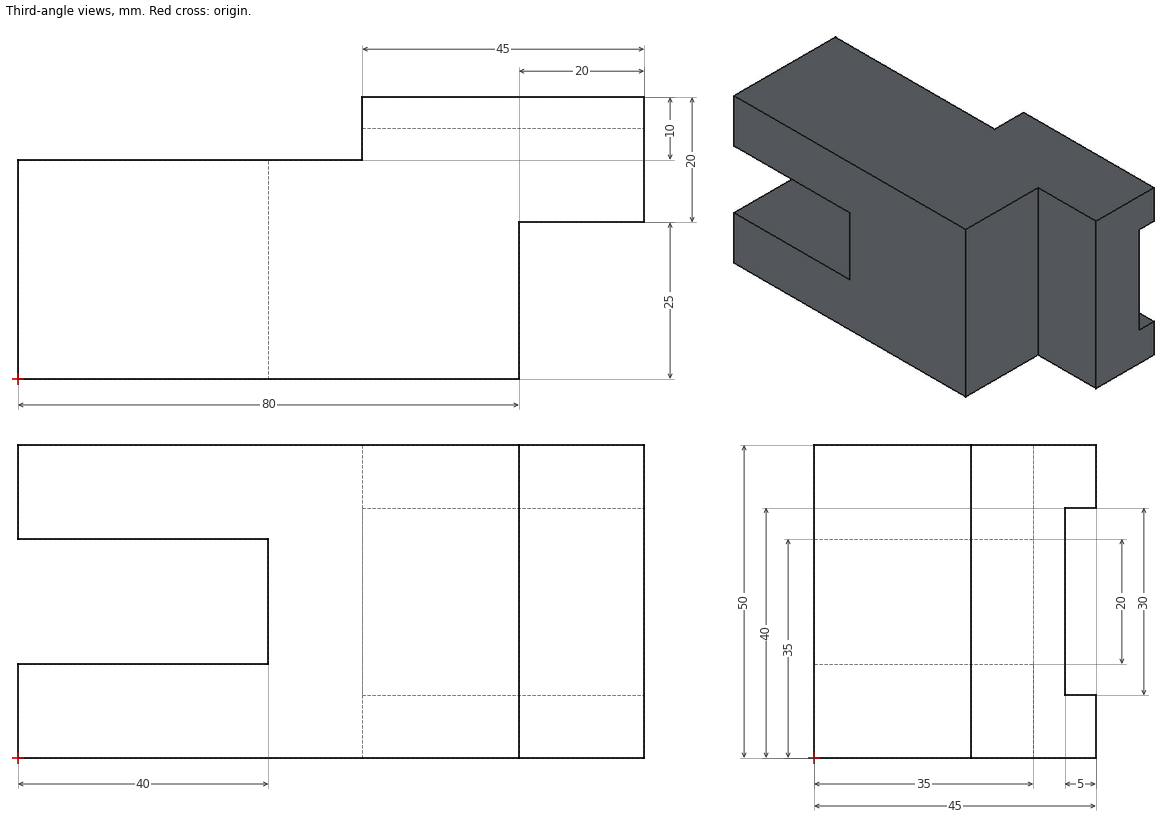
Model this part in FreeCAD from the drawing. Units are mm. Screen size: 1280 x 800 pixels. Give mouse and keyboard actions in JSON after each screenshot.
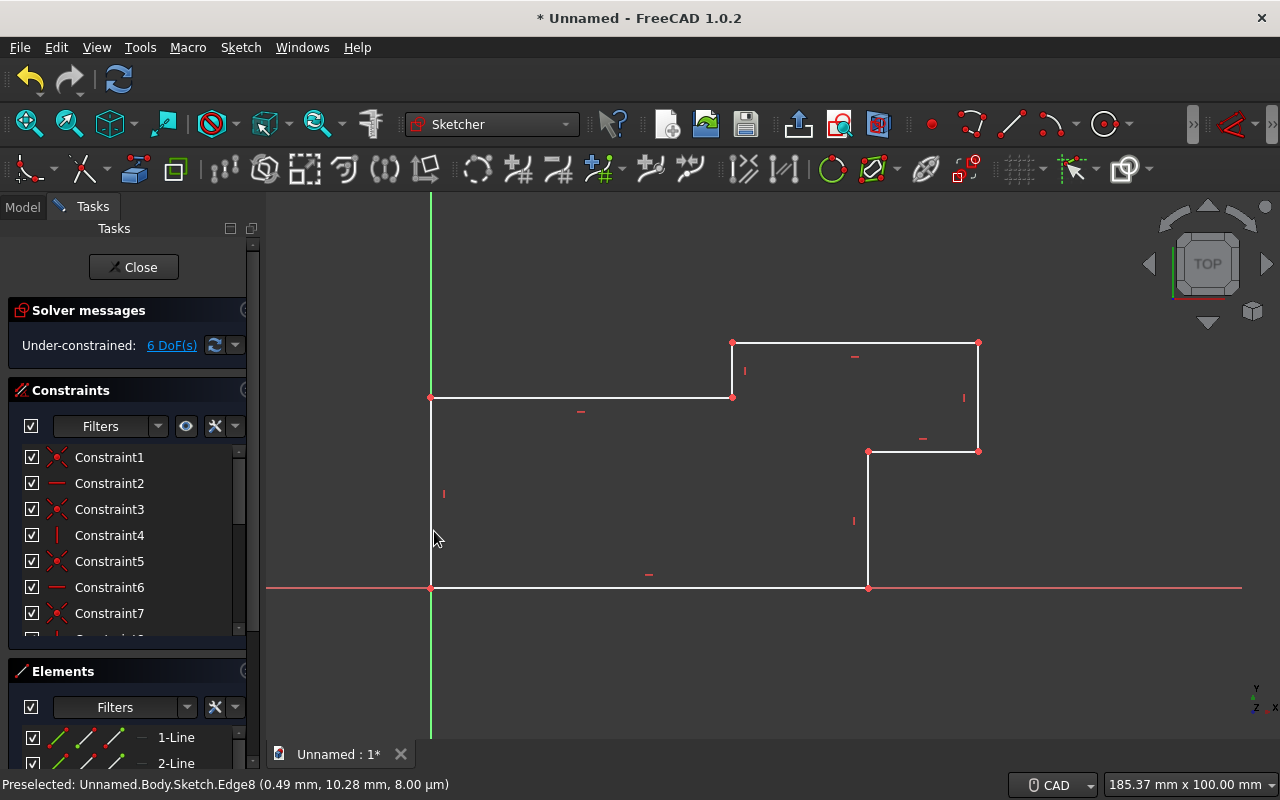
{"action": "left_click", "coordinate": [1232, 124]}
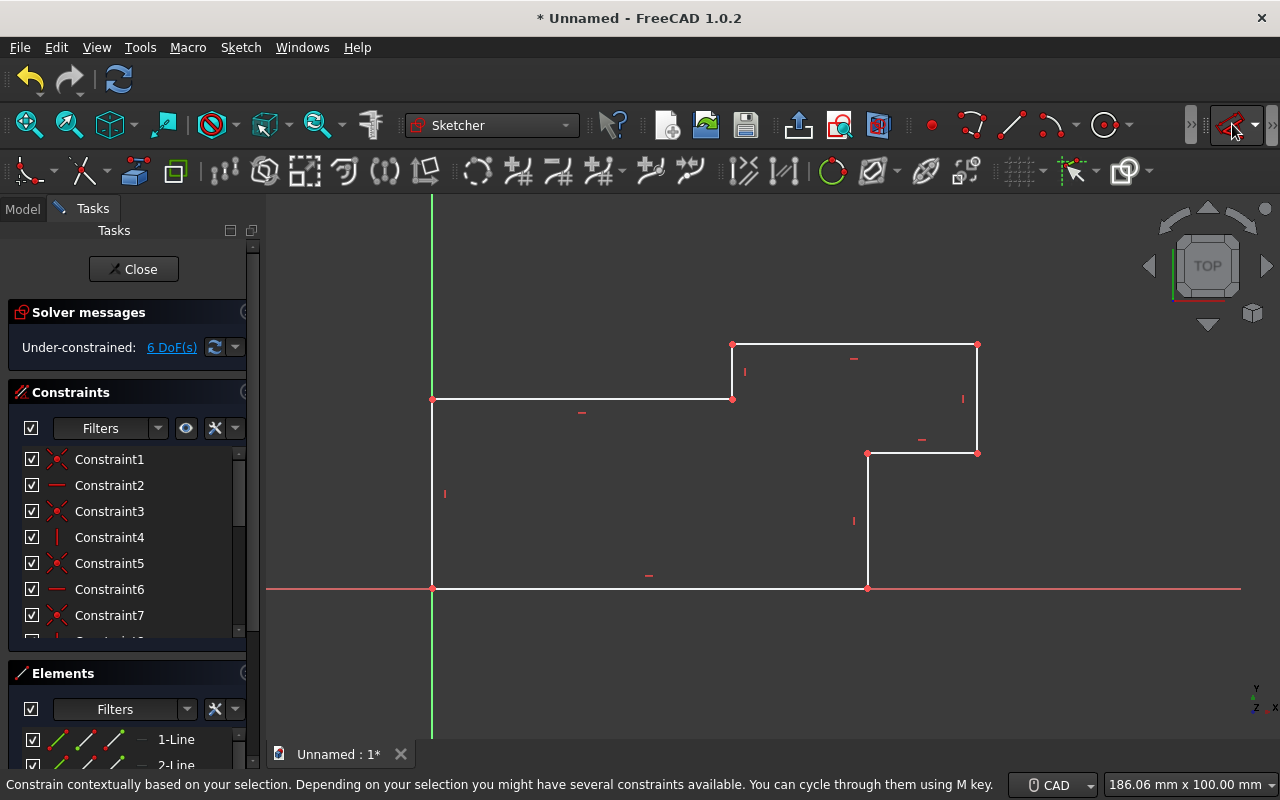
{"action": "left_click", "coordinate": [563, 589]}
{"action": "left_click", "coordinate": [650, 623]}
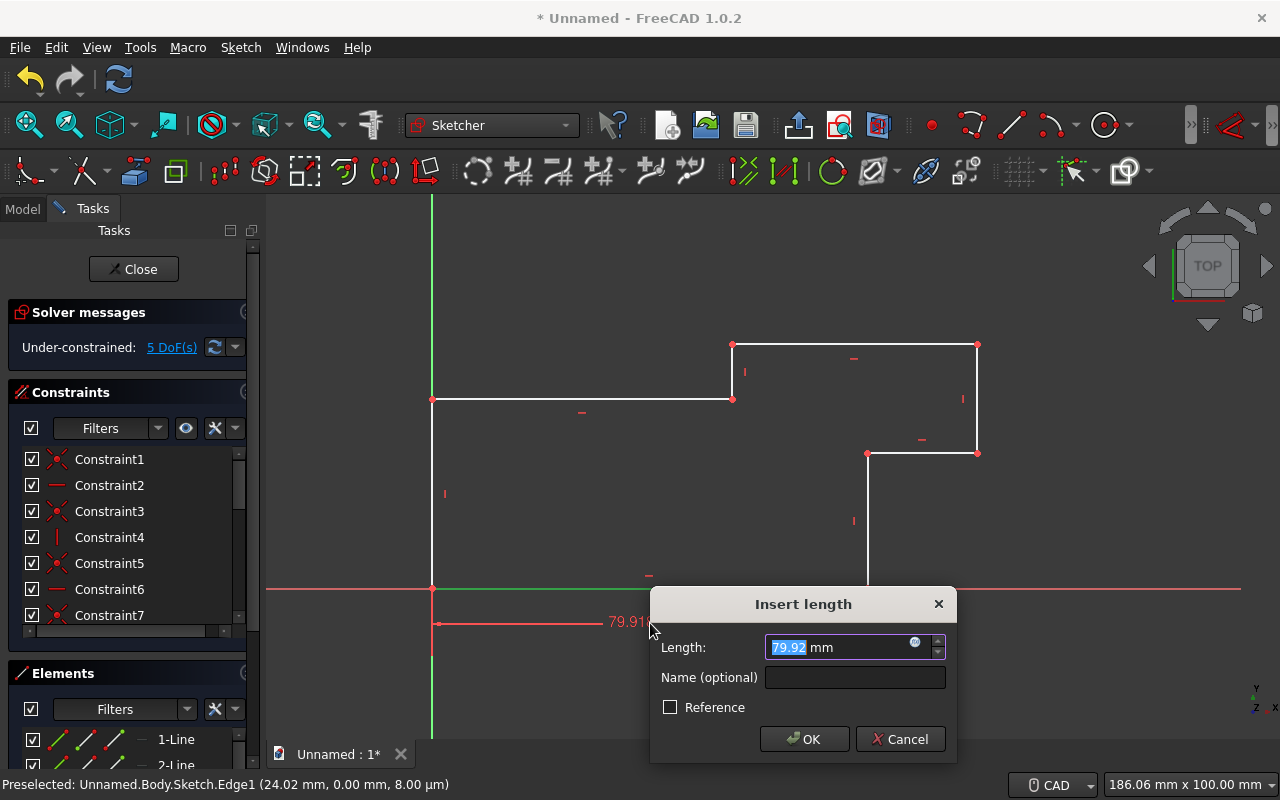
{"action": "type", "text": "80"}
{"action": "key", "text": "Return"}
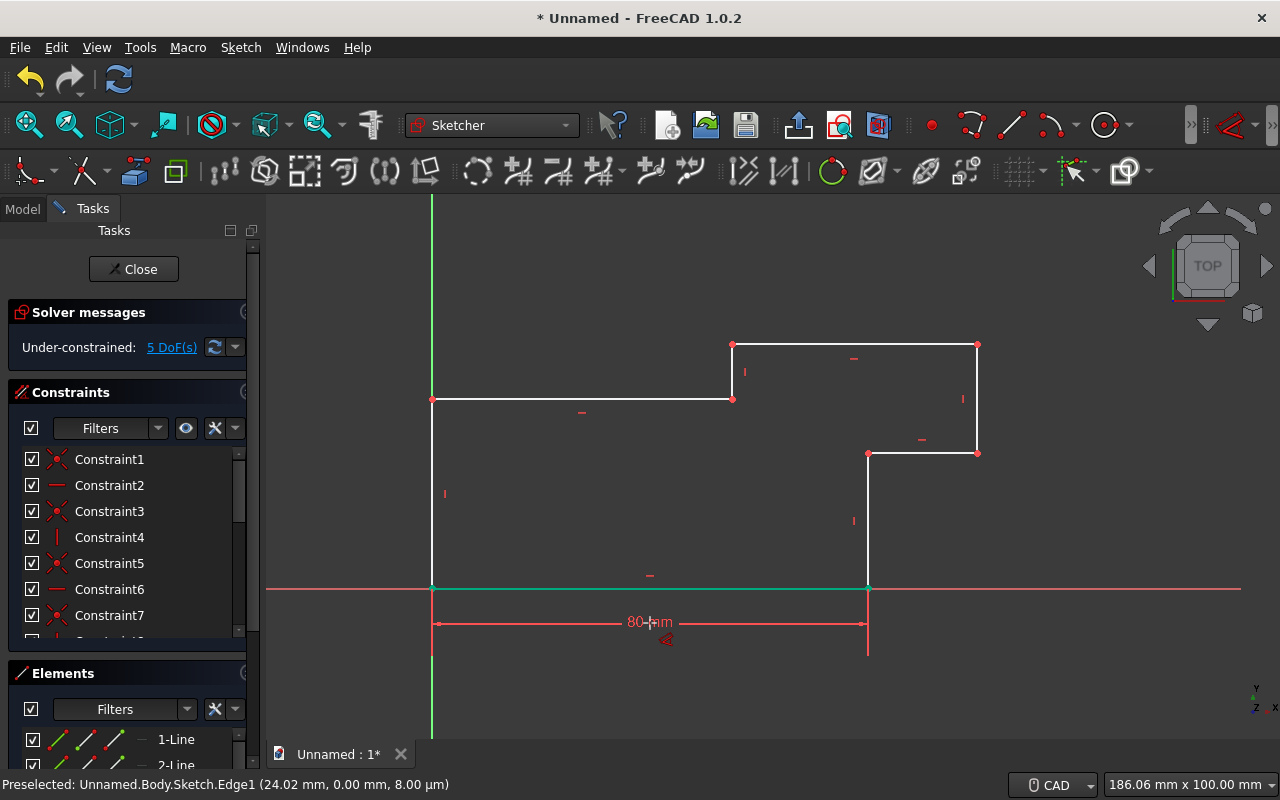
{"action": "left_click", "coordinate": [868, 548]}
{"action": "left_click", "coordinate": [902, 521]}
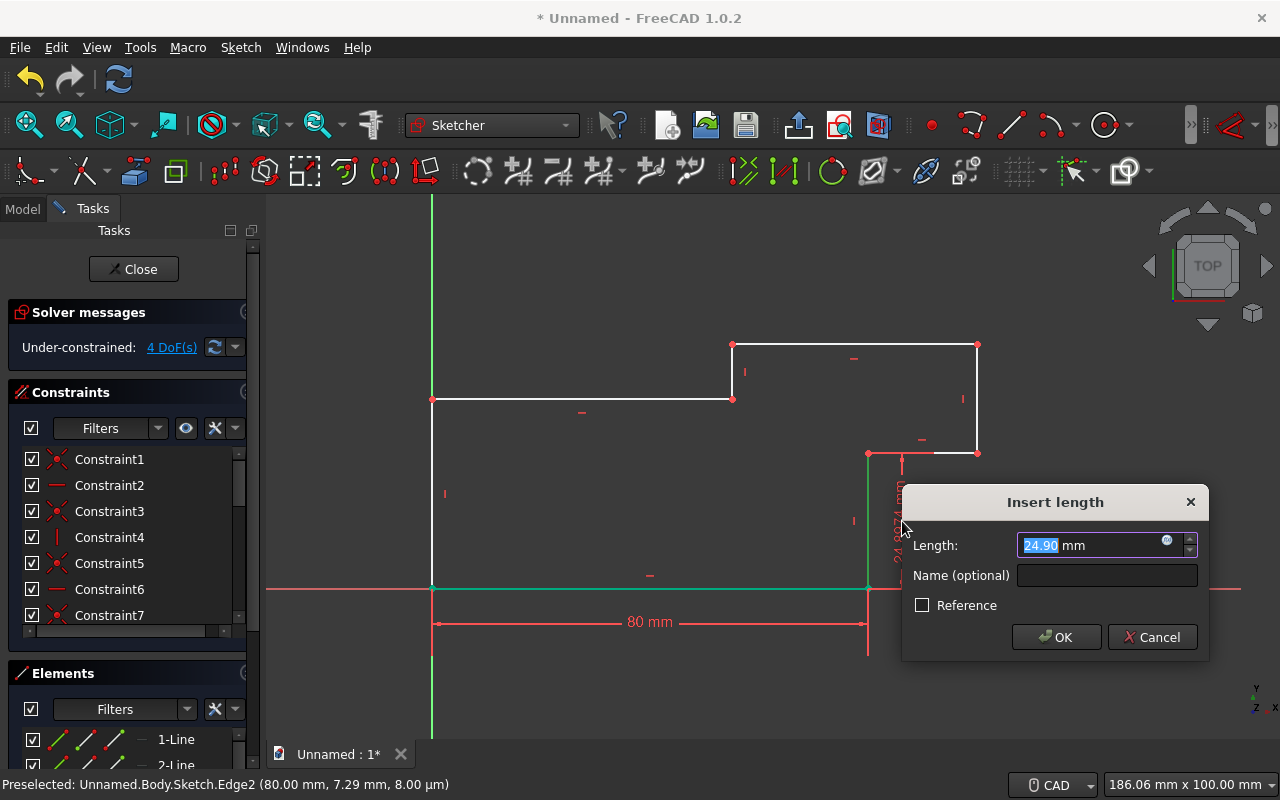
{"action": "type", "text": "25"}
{"action": "key", "text": "Return"}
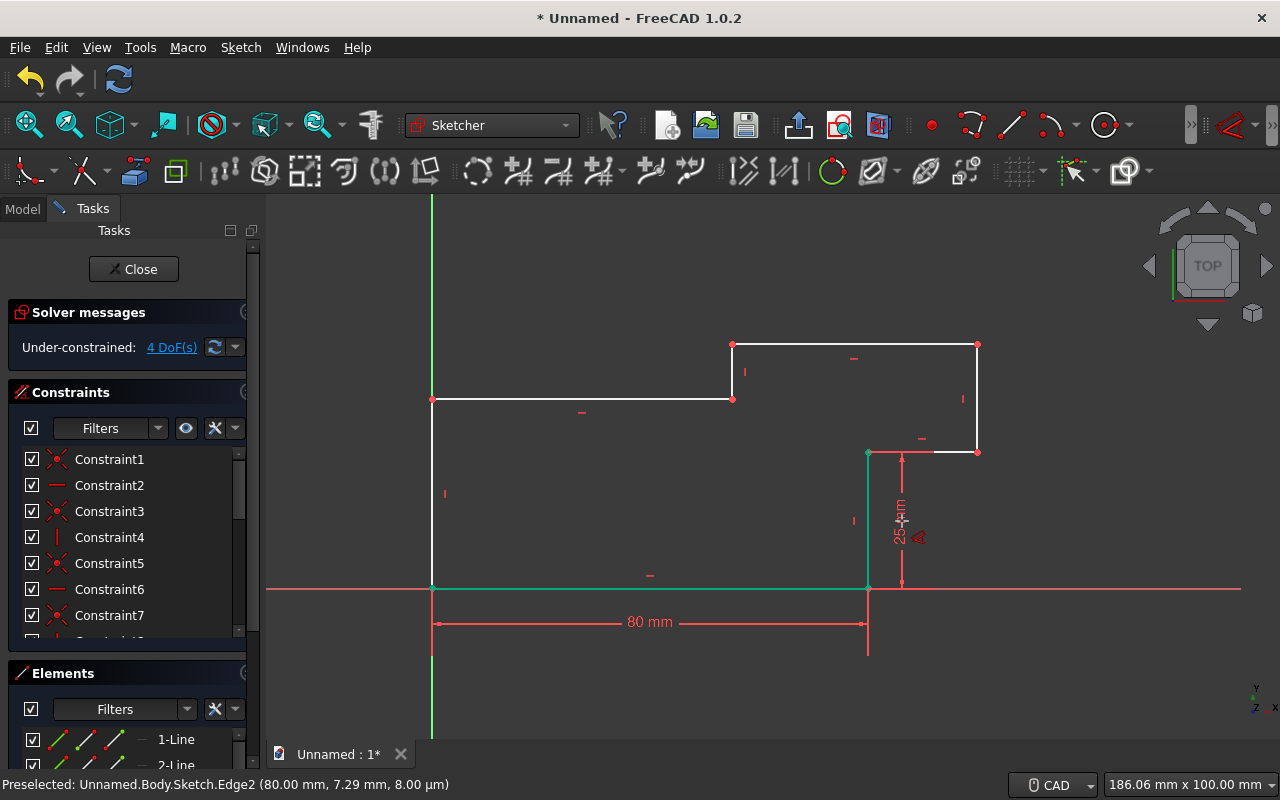
{"action": "left_click", "coordinate": [901, 452]}
{"action": "left_click", "coordinate": [923, 418]}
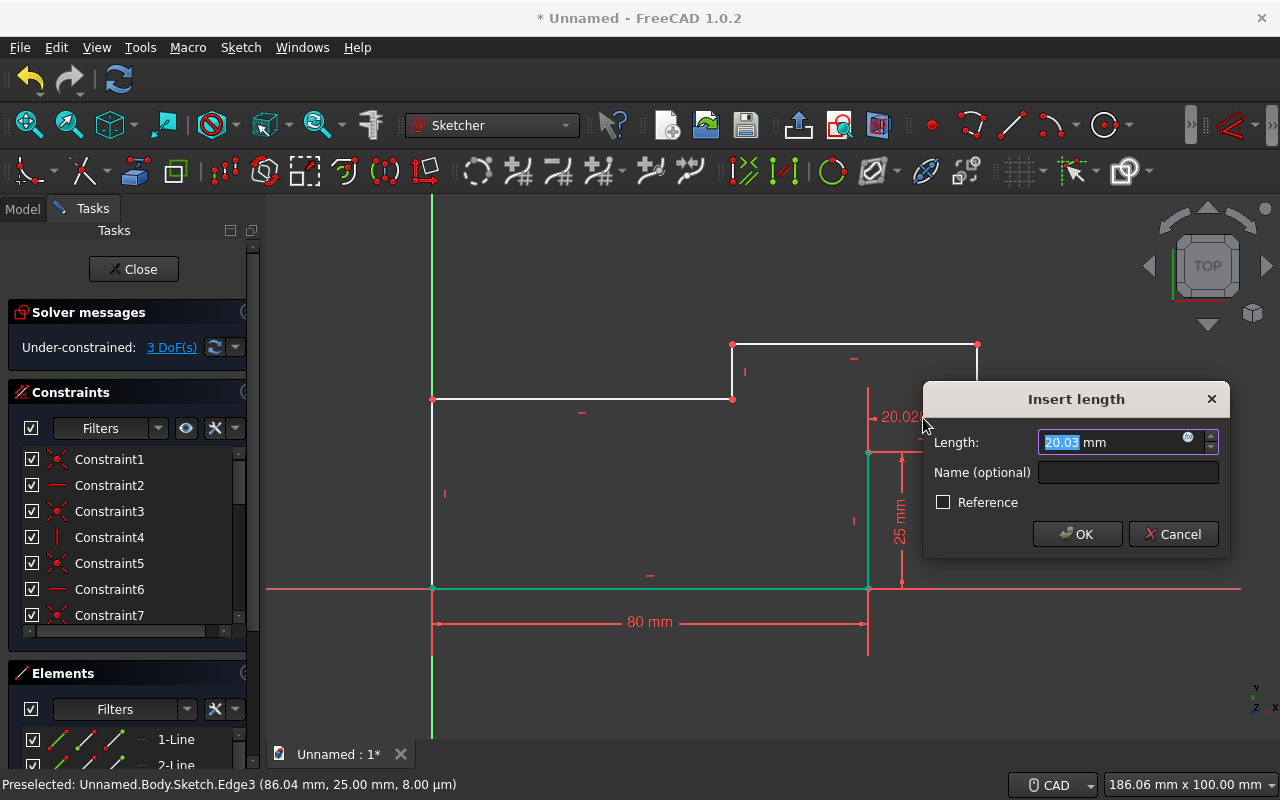
{"action": "type", "text": "20"}
{"action": "key", "text": "Return"}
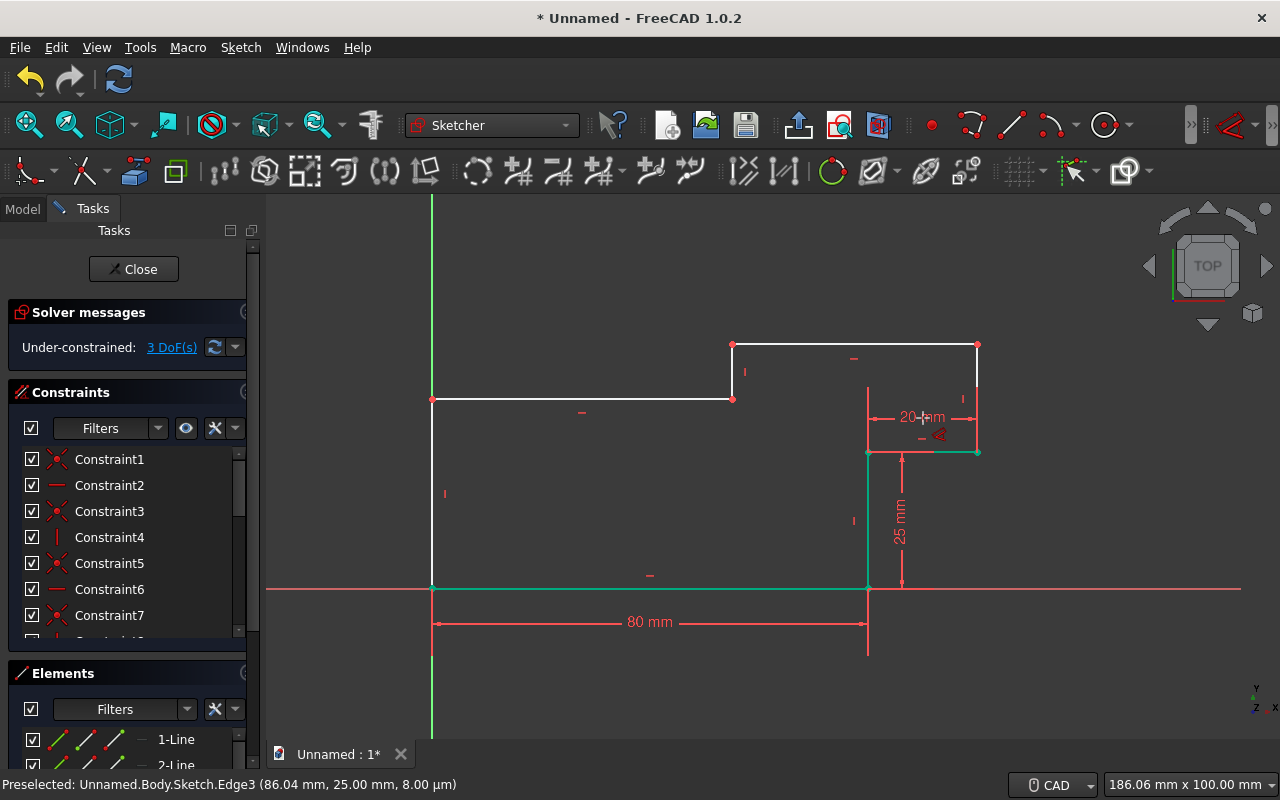
{"action": "left_click", "coordinate": [977, 420]}
{"action": "left_click", "coordinate": [1011, 398]}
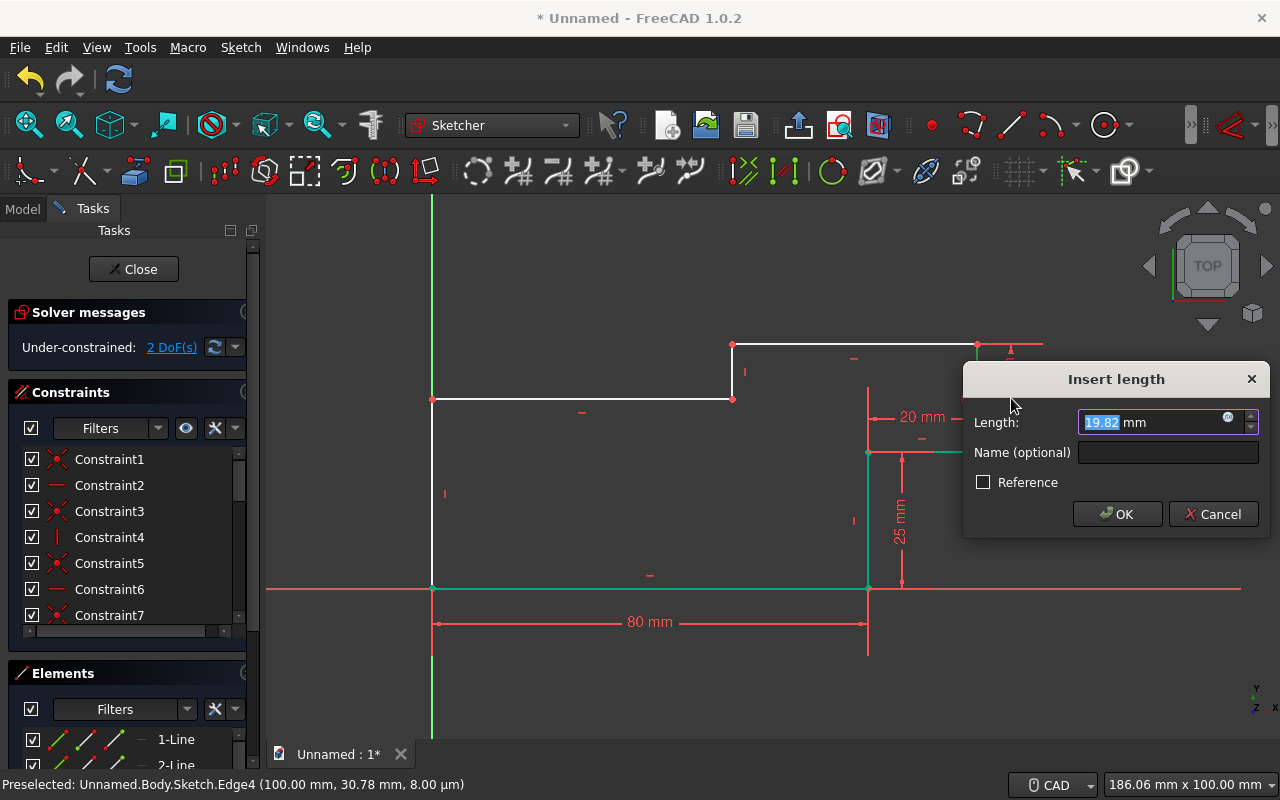
{"action": "type", "text": "20"}
{"action": "key", "text": "Return"}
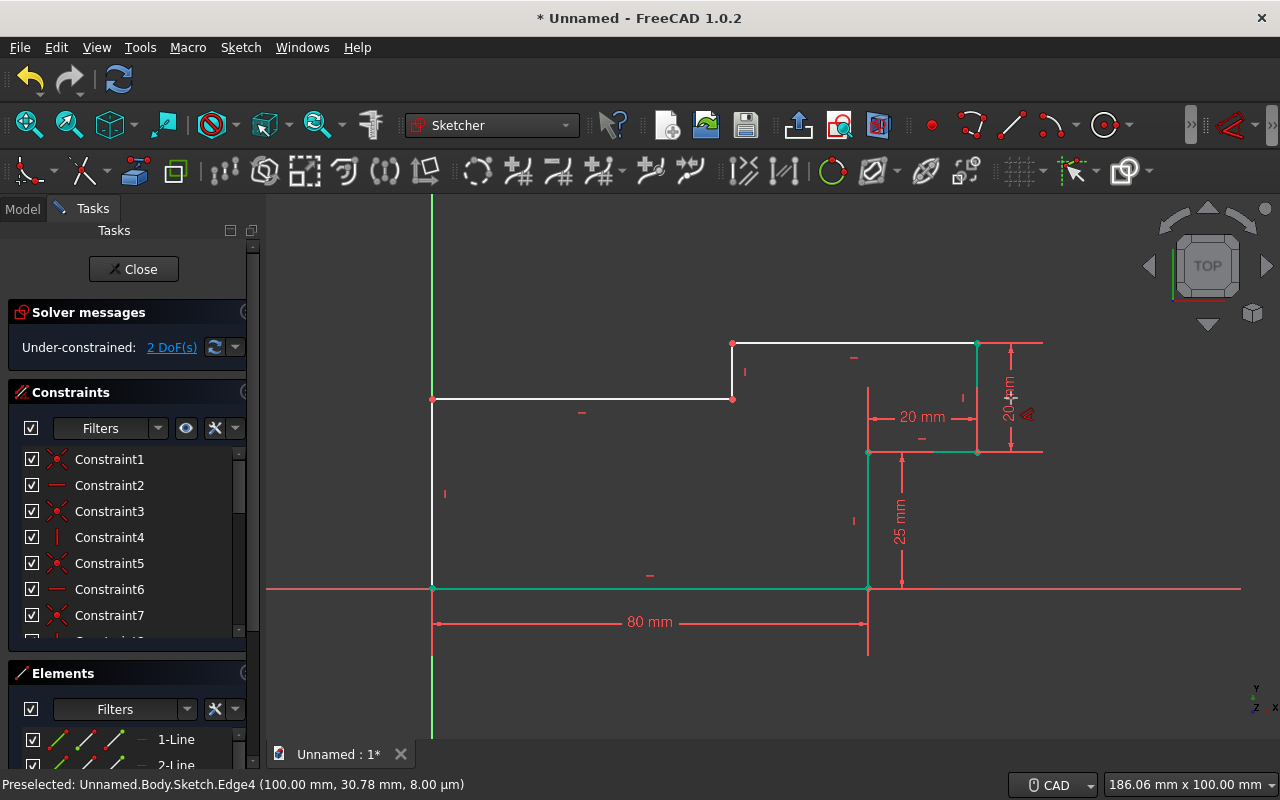
{"action": "left_click", "coordinate": [904, 343]}
{"action": "left_click", "coordinate": [855, 309]}